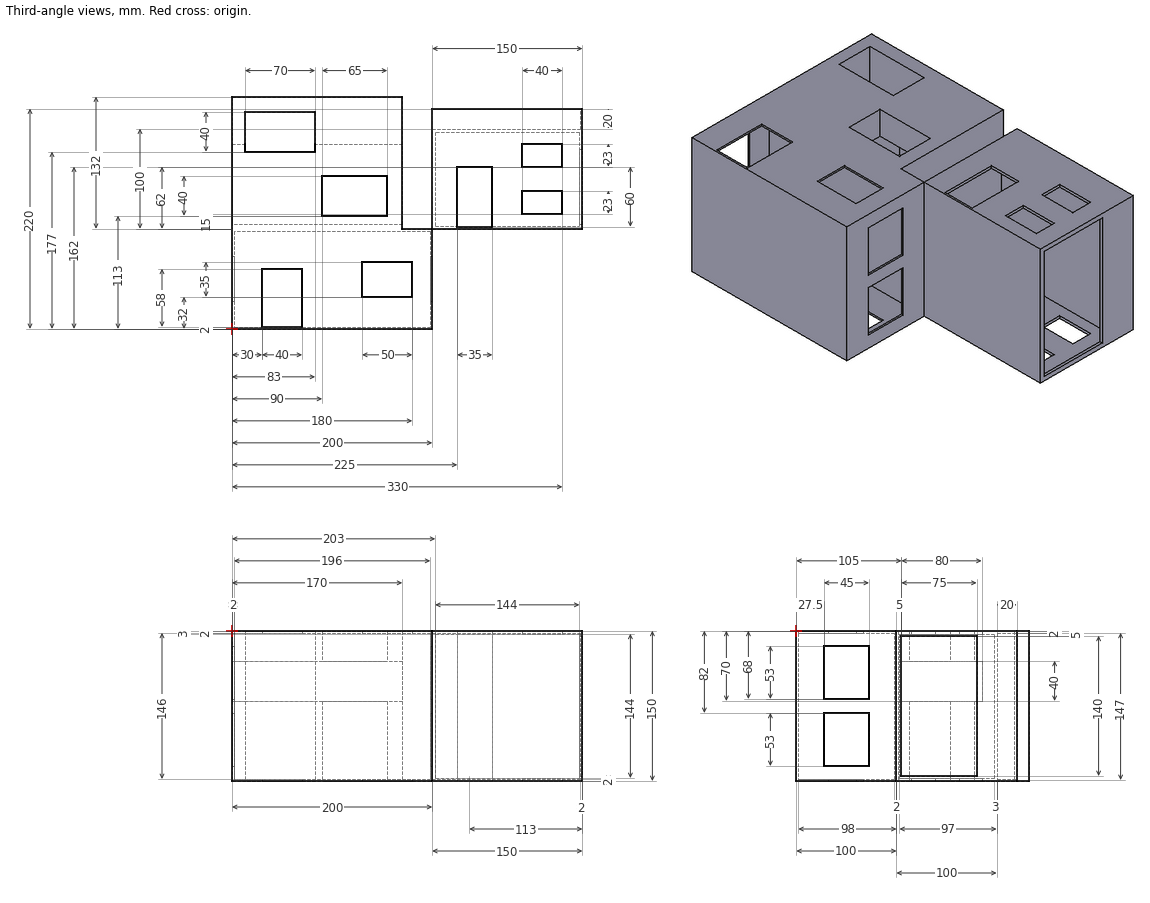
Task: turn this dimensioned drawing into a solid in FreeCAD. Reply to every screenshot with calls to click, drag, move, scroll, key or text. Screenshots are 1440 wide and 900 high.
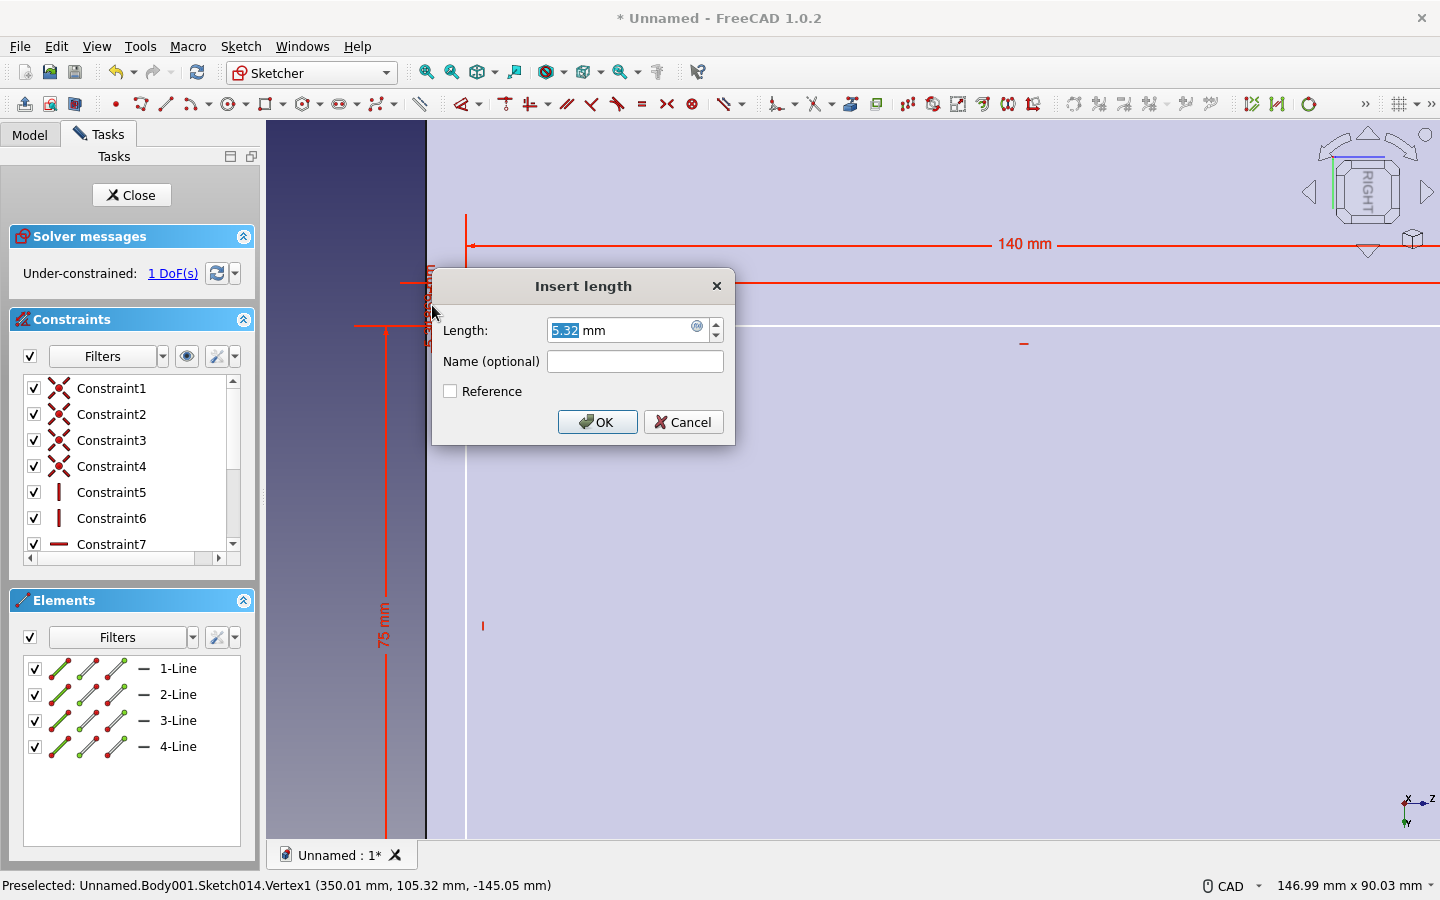
text(5)
key(Return)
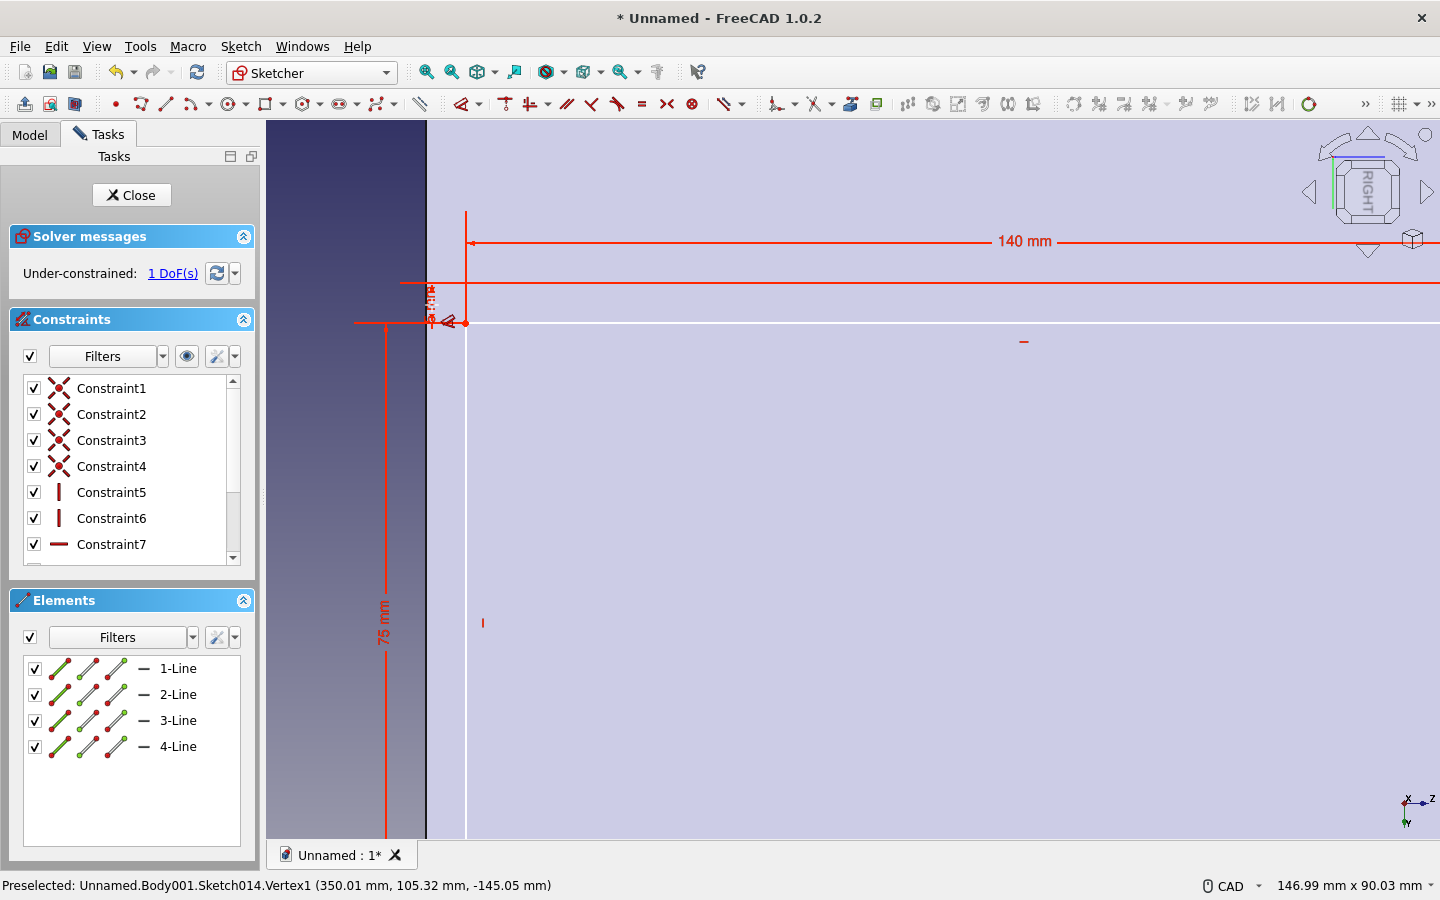
scroll(467, 330, down, 3)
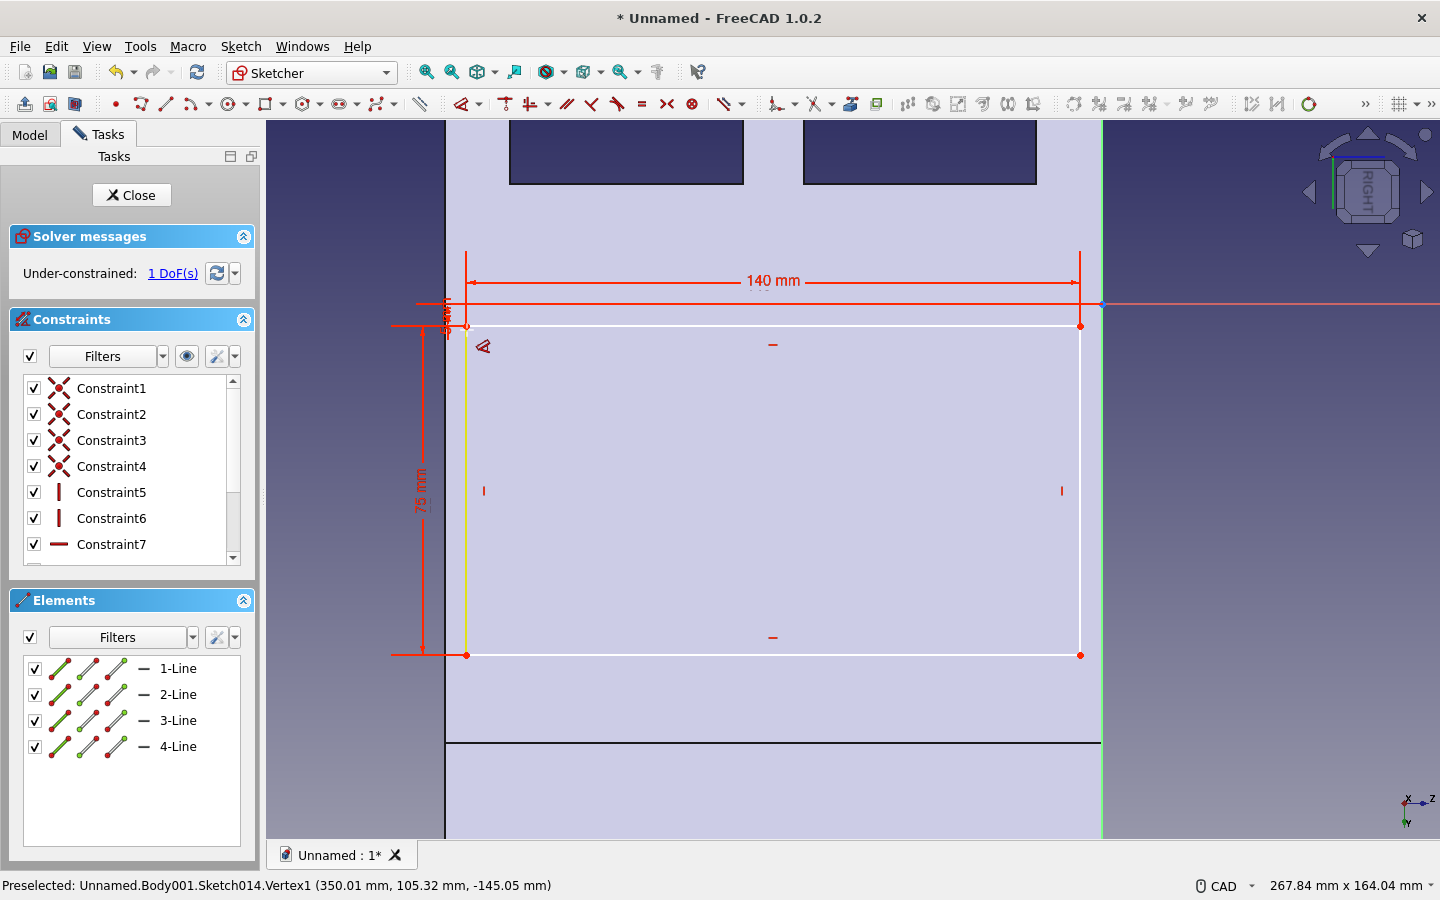
scroll(1080, 655, up, 3)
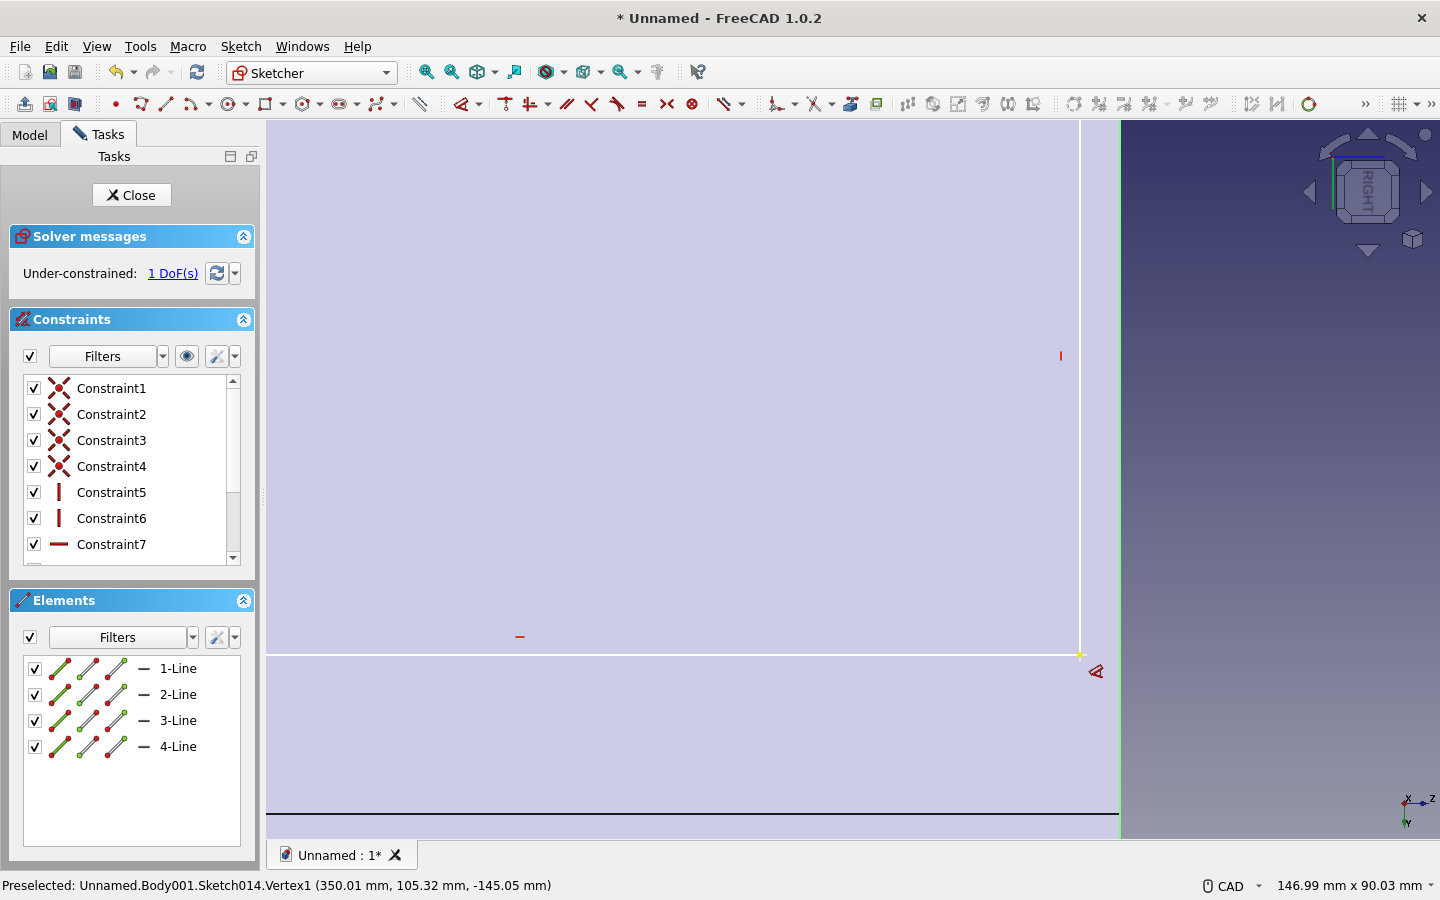
click(1080, 655)
click(1100, 689)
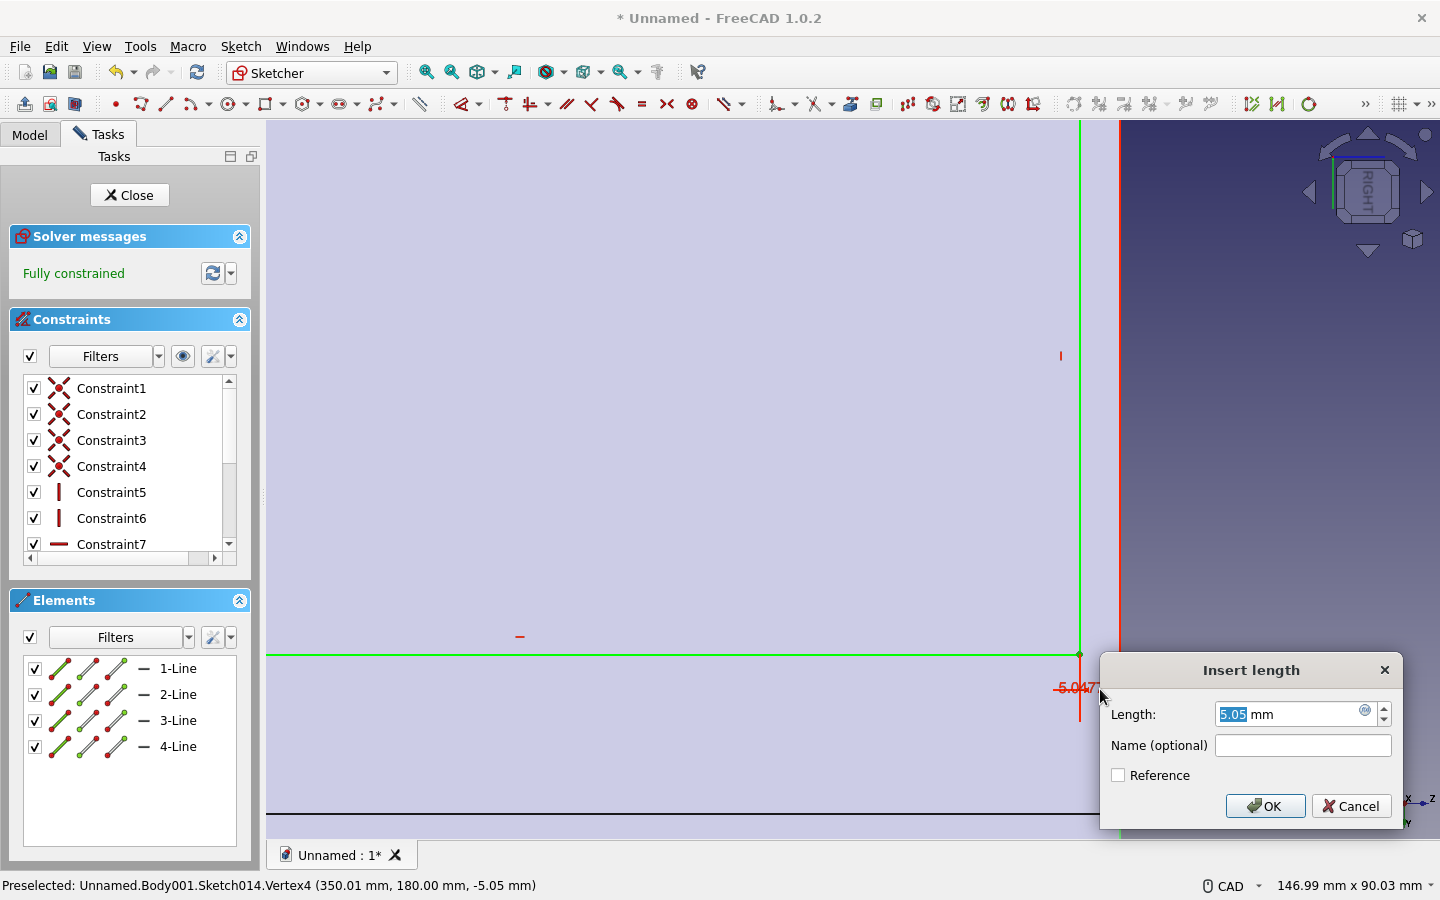
text(5)
key(Return)
key(Escape)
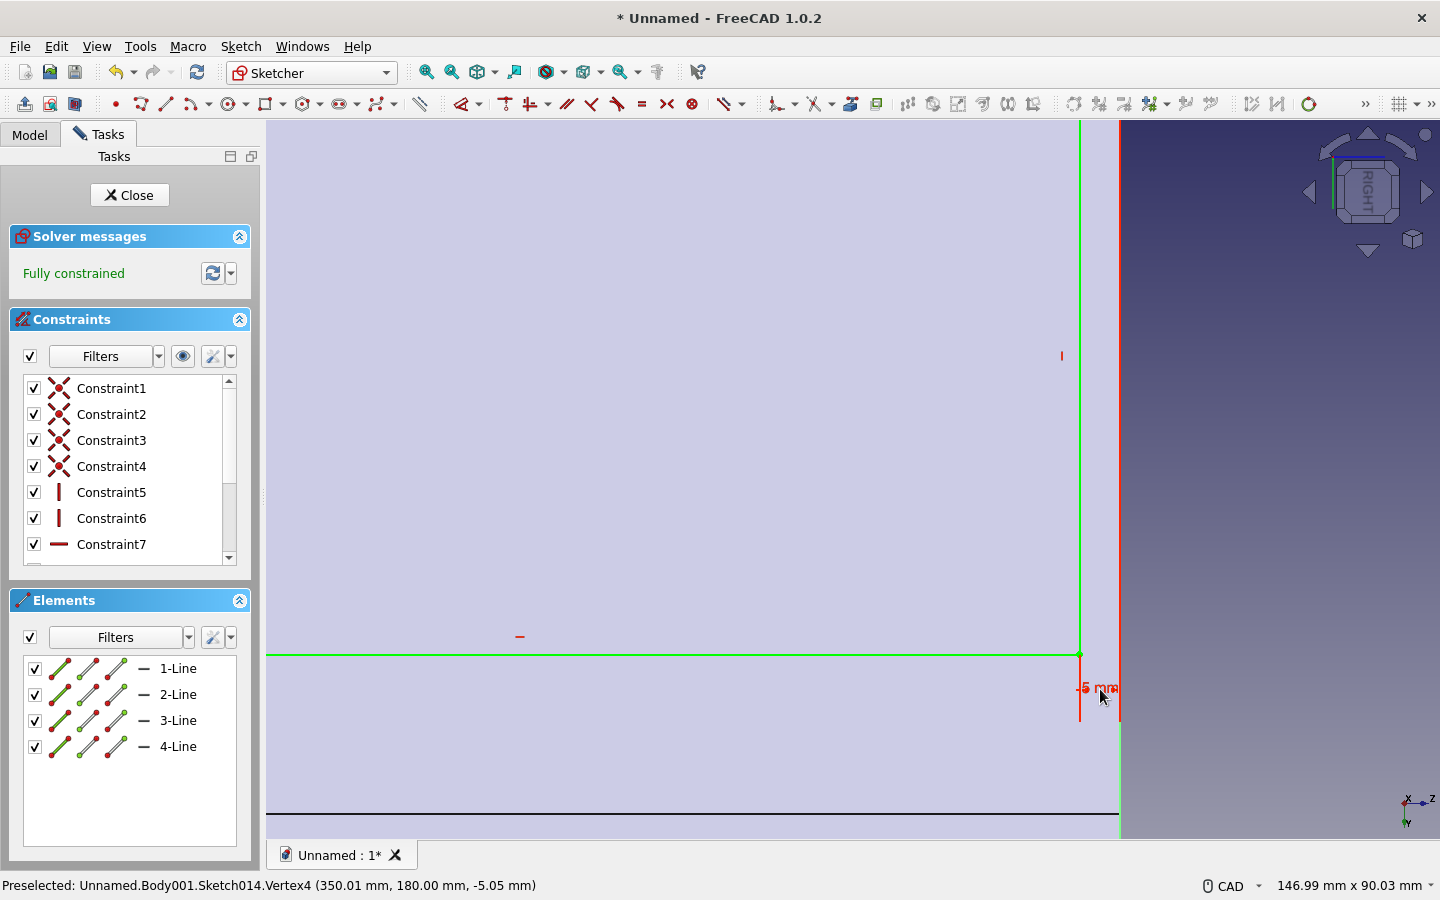
click(130, 195)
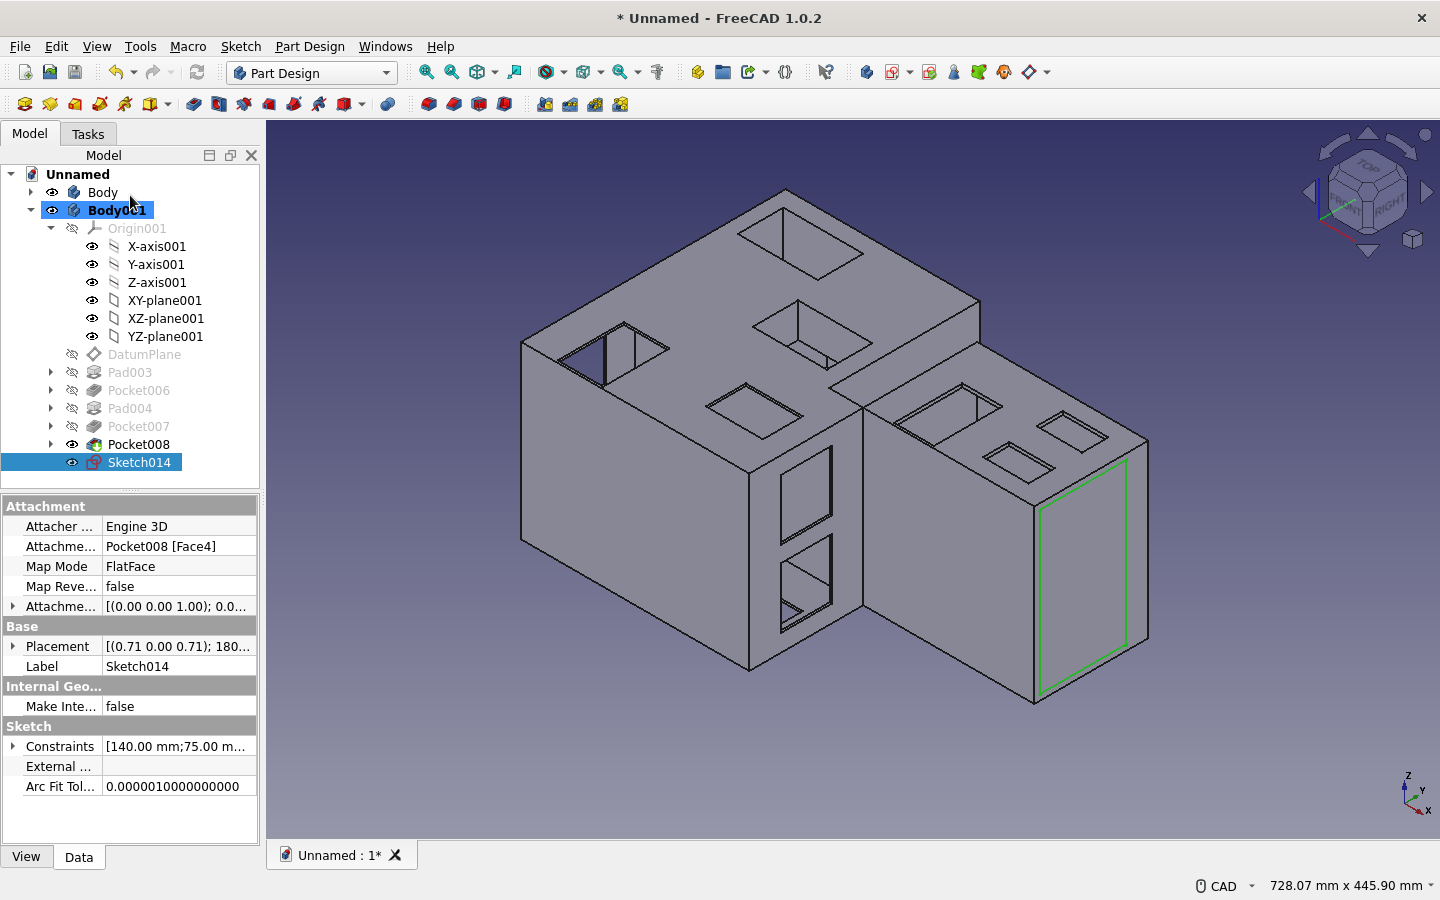
click(194, 104)